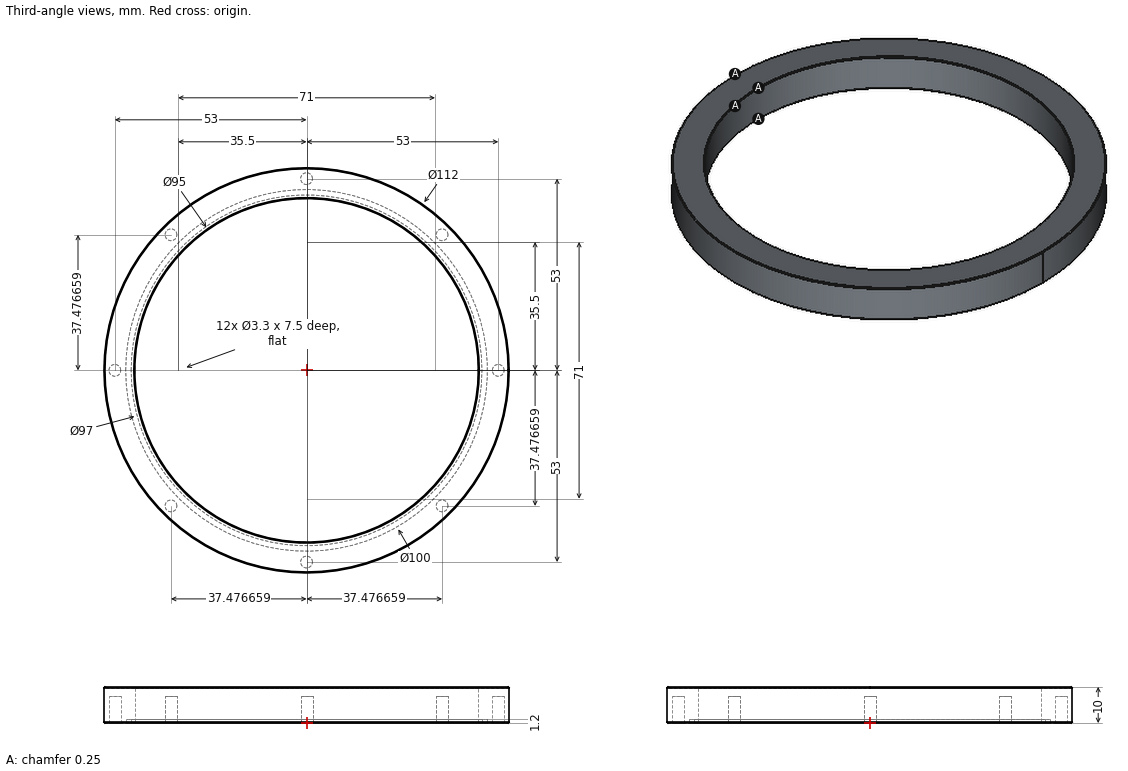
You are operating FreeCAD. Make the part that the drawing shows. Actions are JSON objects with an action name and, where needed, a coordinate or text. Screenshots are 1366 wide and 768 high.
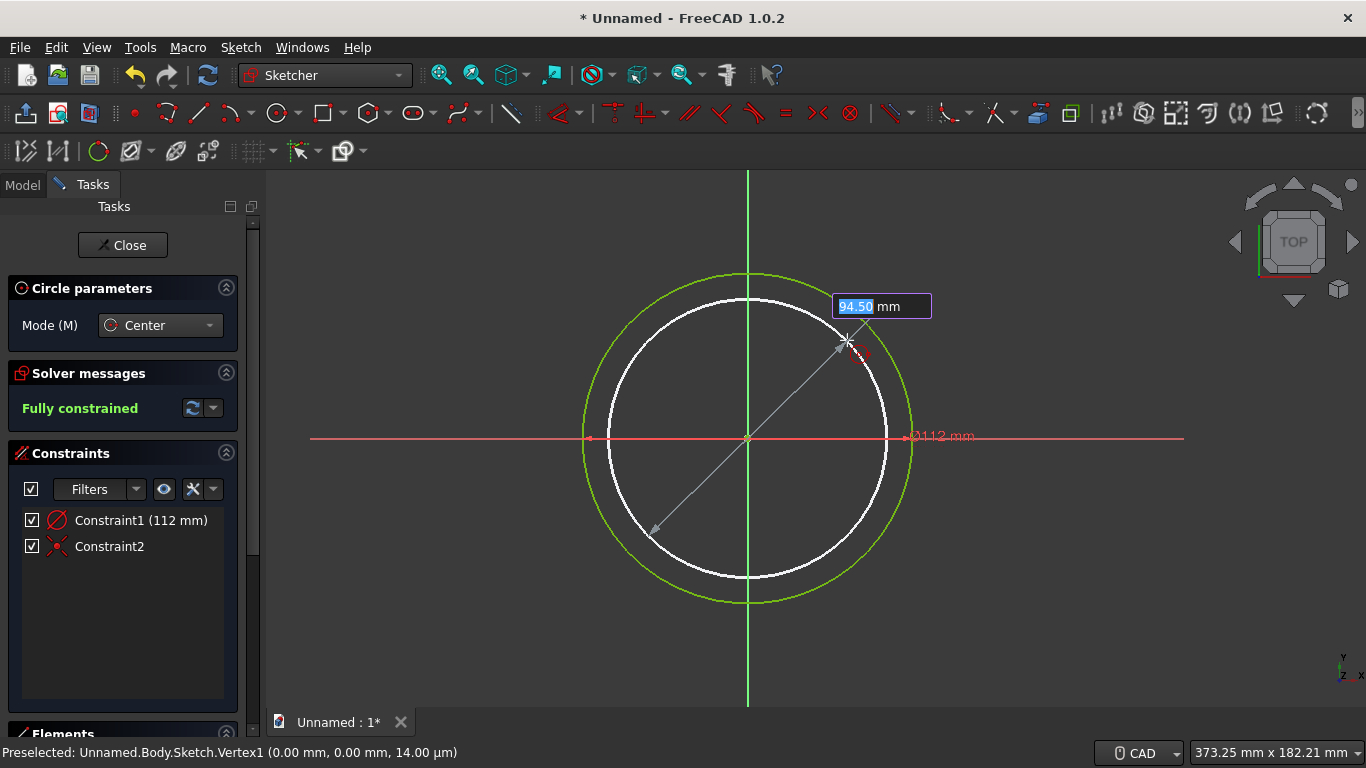
{"action": "type", "text": "95"}
{"action": "key", "text": "Return"}
{"action": "key", "text": "Escape"}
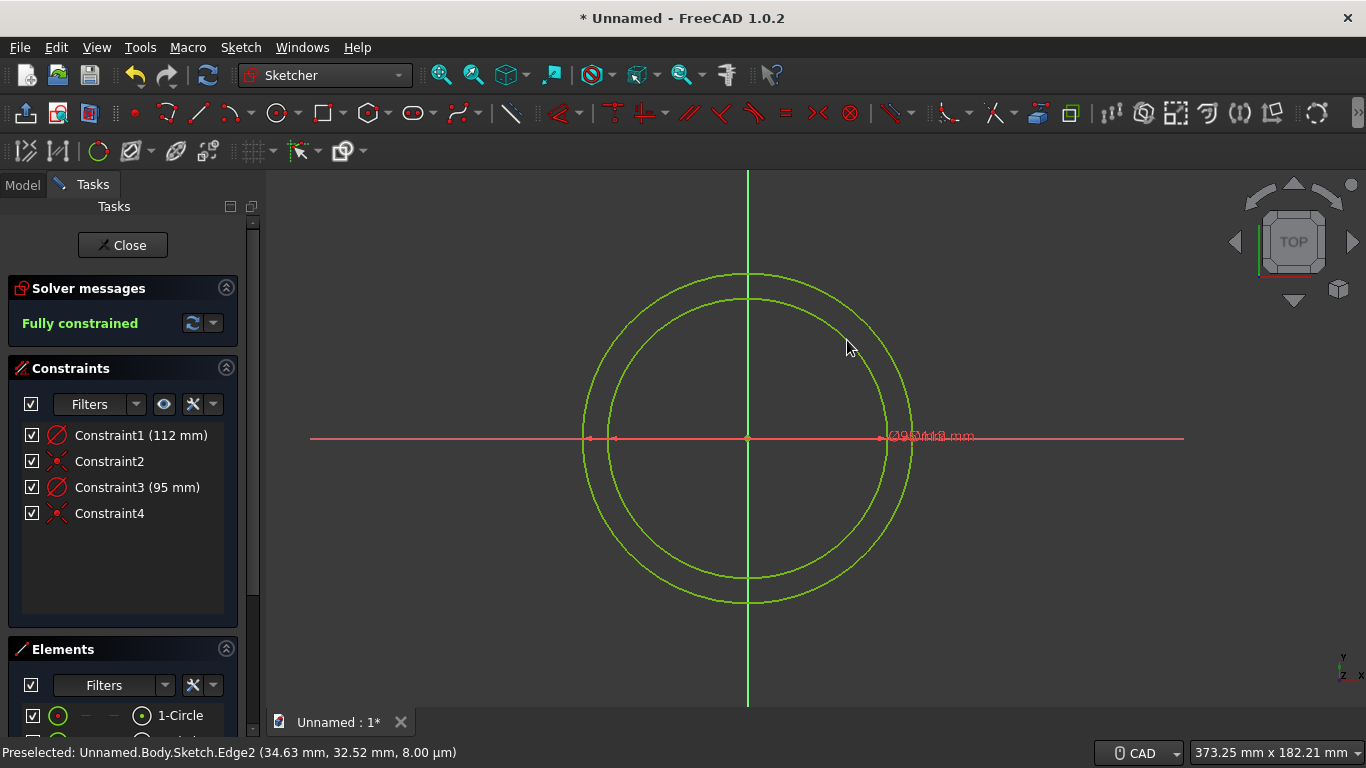
{"action": "left_click", "coordinate": [123, 245]}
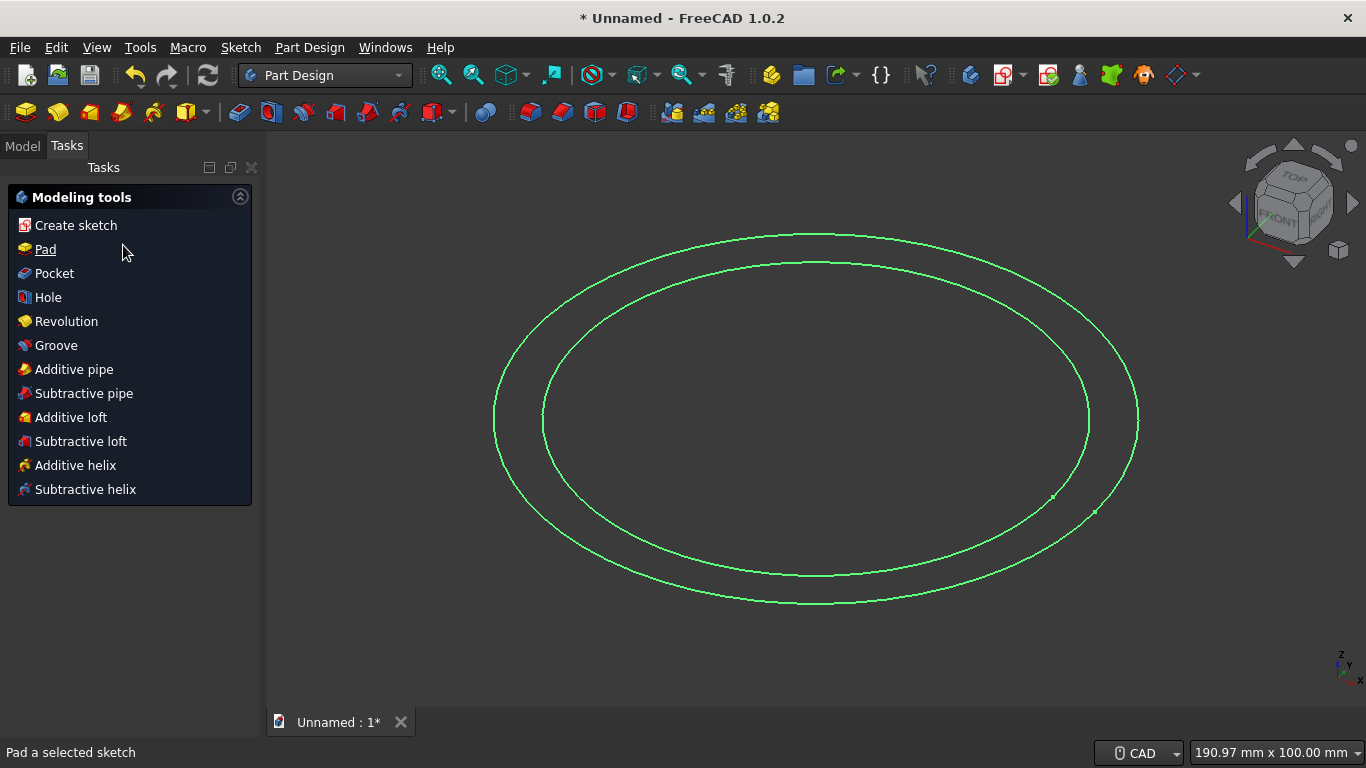
{"action": "left_click", "coordinate": [26, 112]}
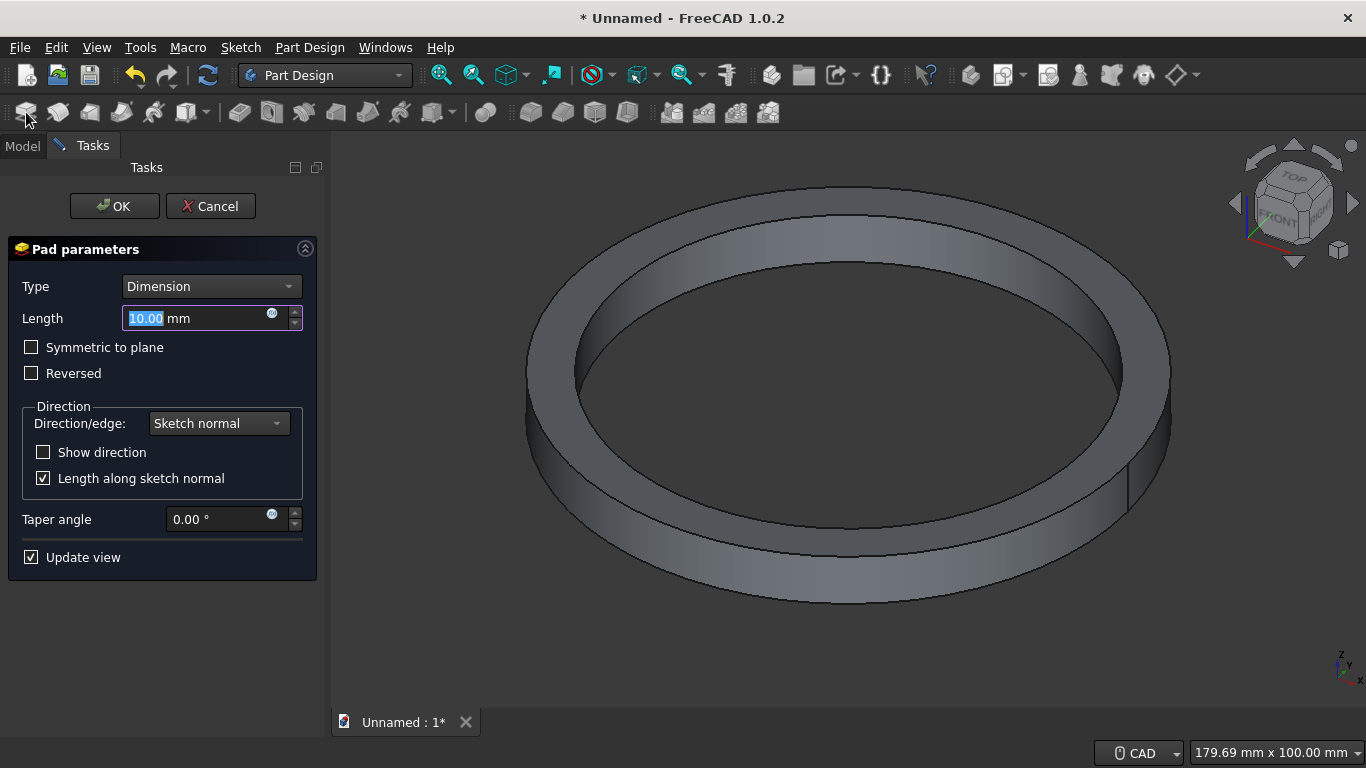
{"action": "type", "text": "10"}
{"action": "key", "text": "Tab"}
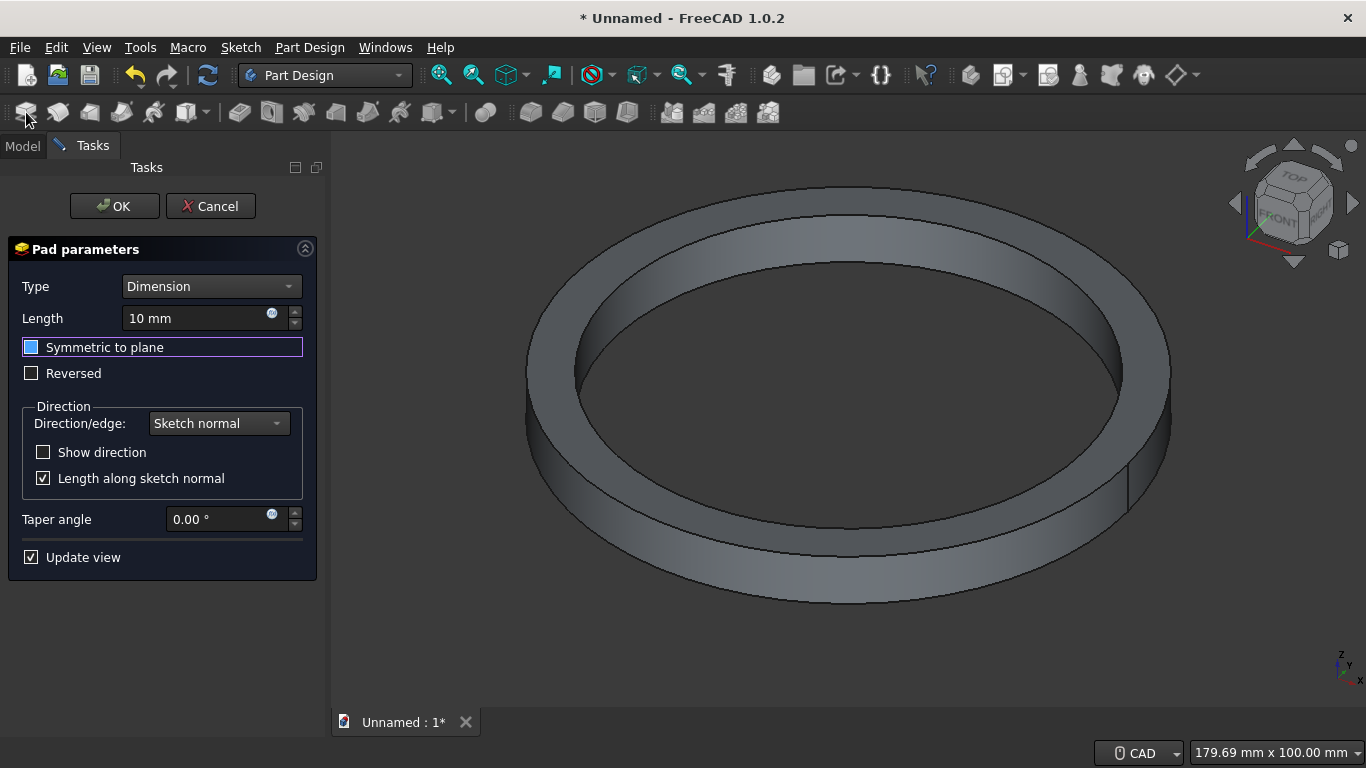
{"action": "left_click", "coordinate": [115, 206]}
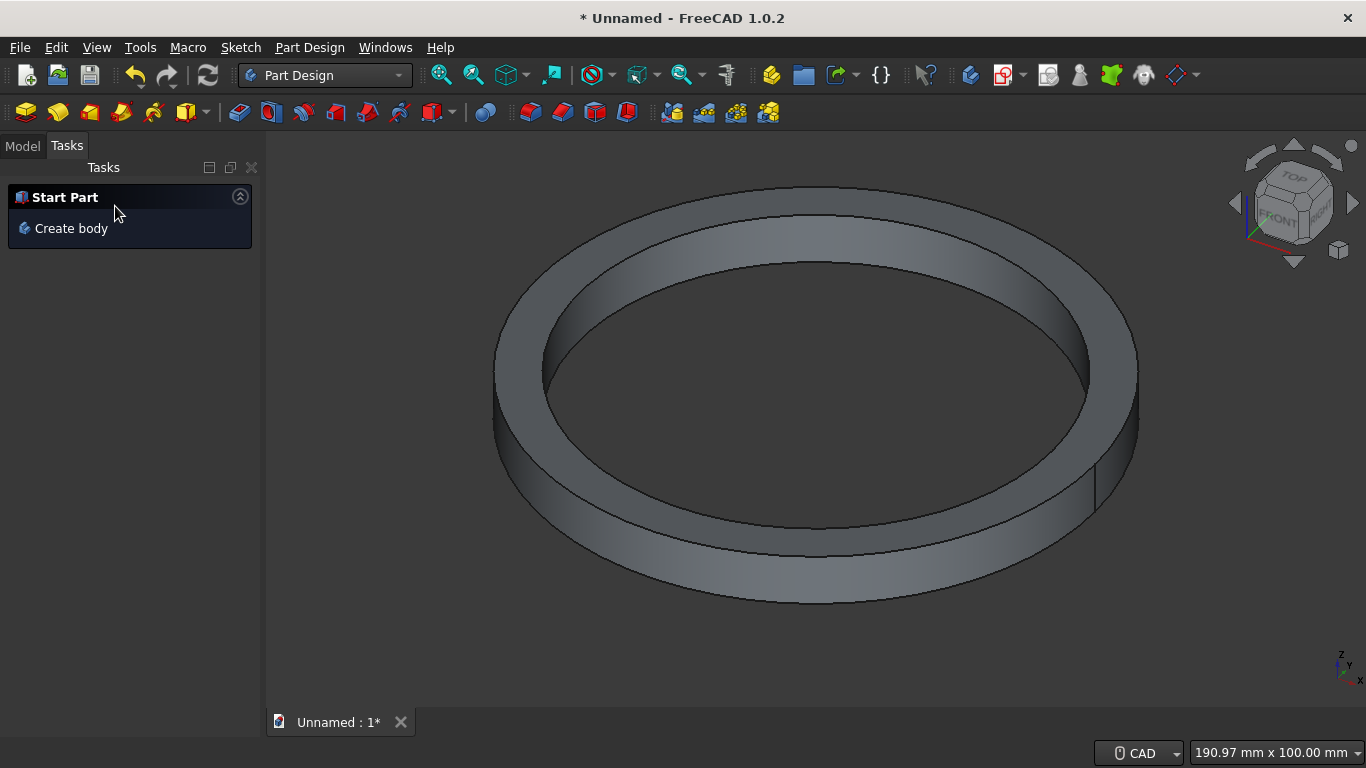
{"action": "left_click", "coordinate": [442, 76]}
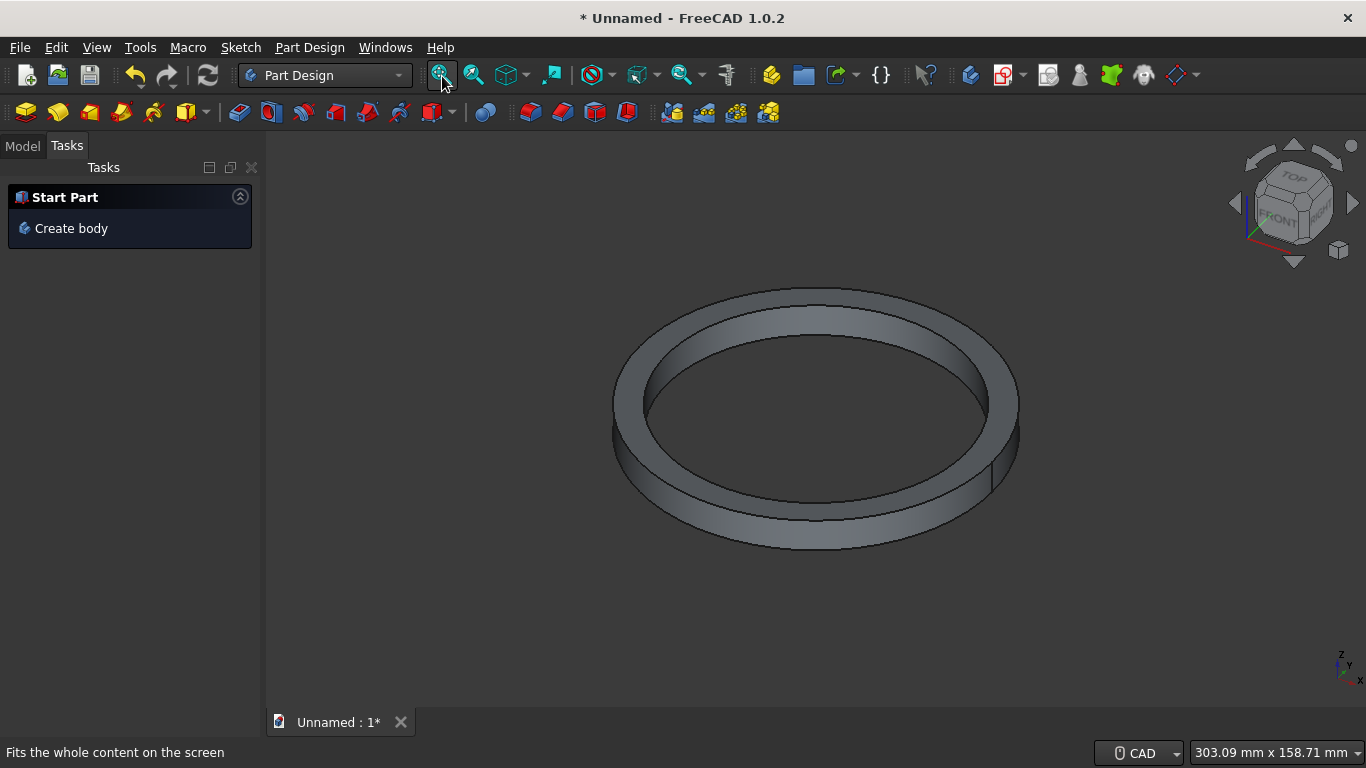
{"action": "left_click", "coordinate": [1004, 76]}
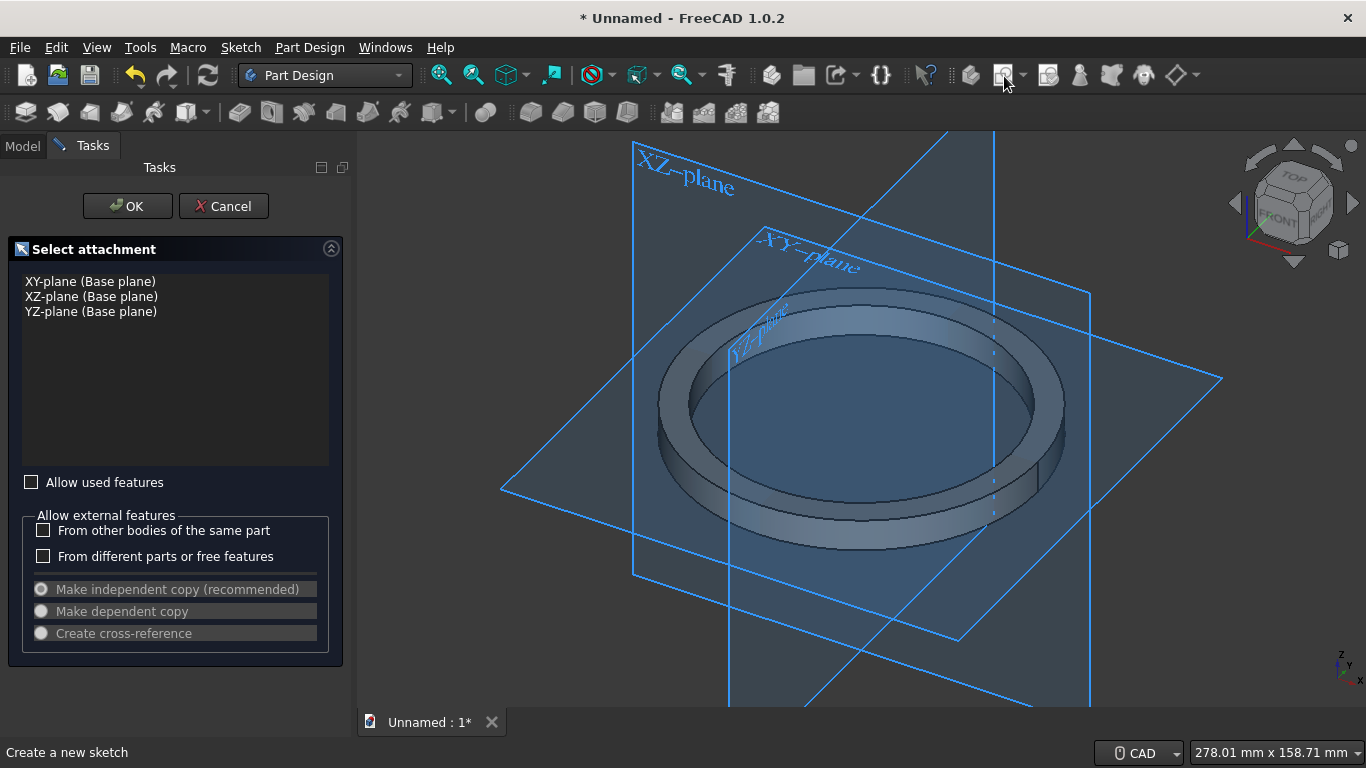
{"action": "left_click", "coordinate": [82, 282]}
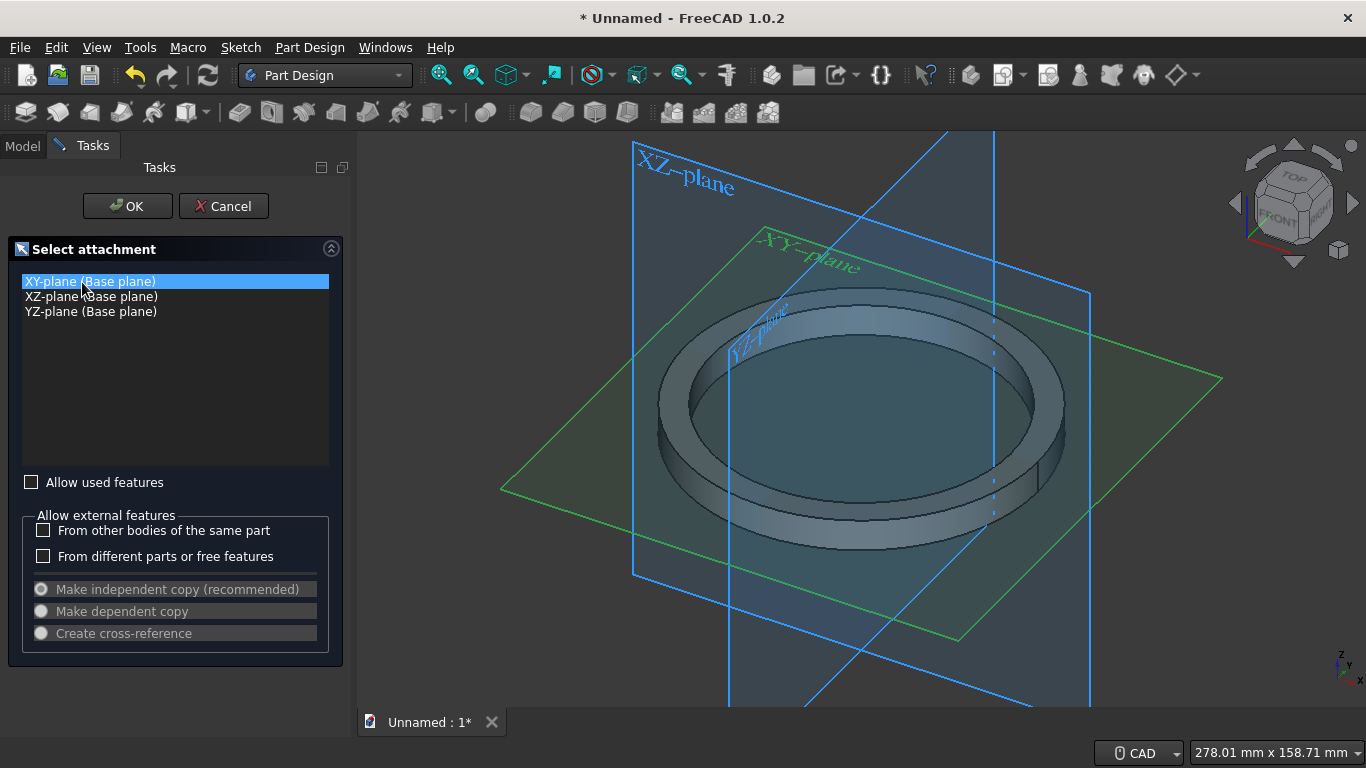
{"action": "left_click", "coordinate": [128, 206]}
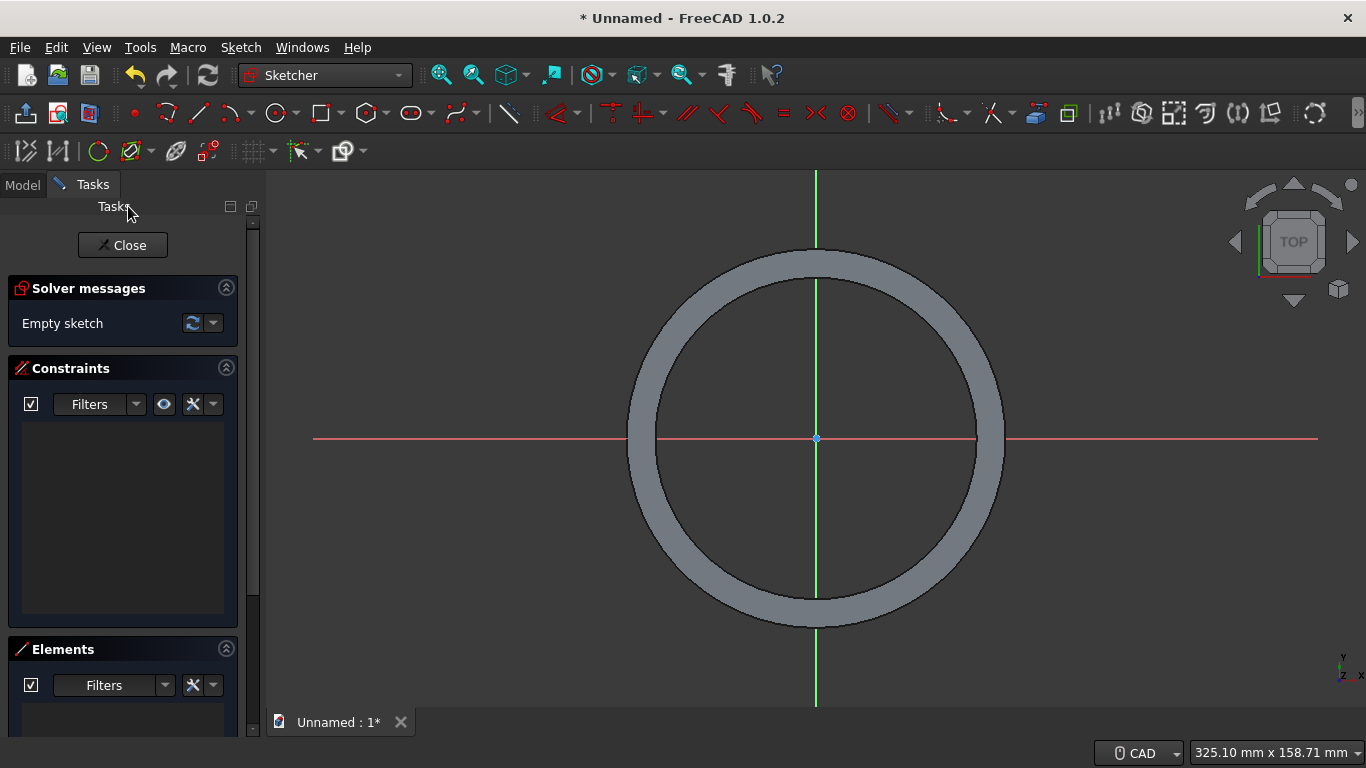
{"action": "key", "text": "q s"}